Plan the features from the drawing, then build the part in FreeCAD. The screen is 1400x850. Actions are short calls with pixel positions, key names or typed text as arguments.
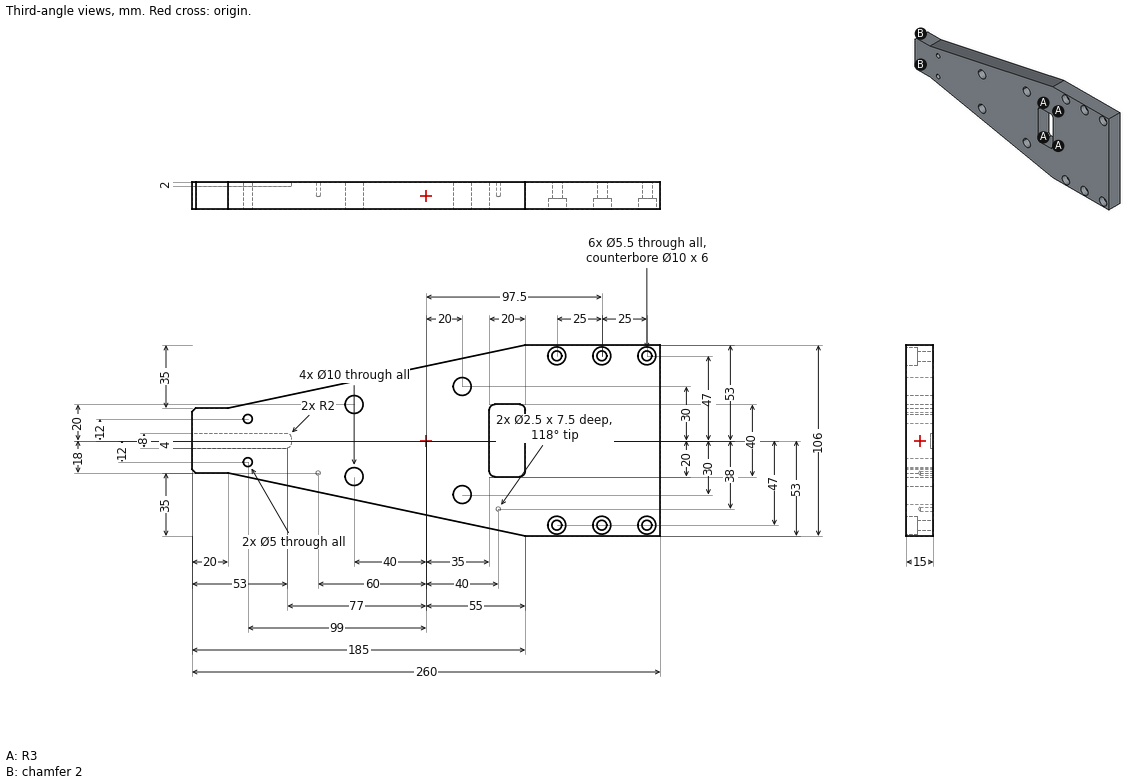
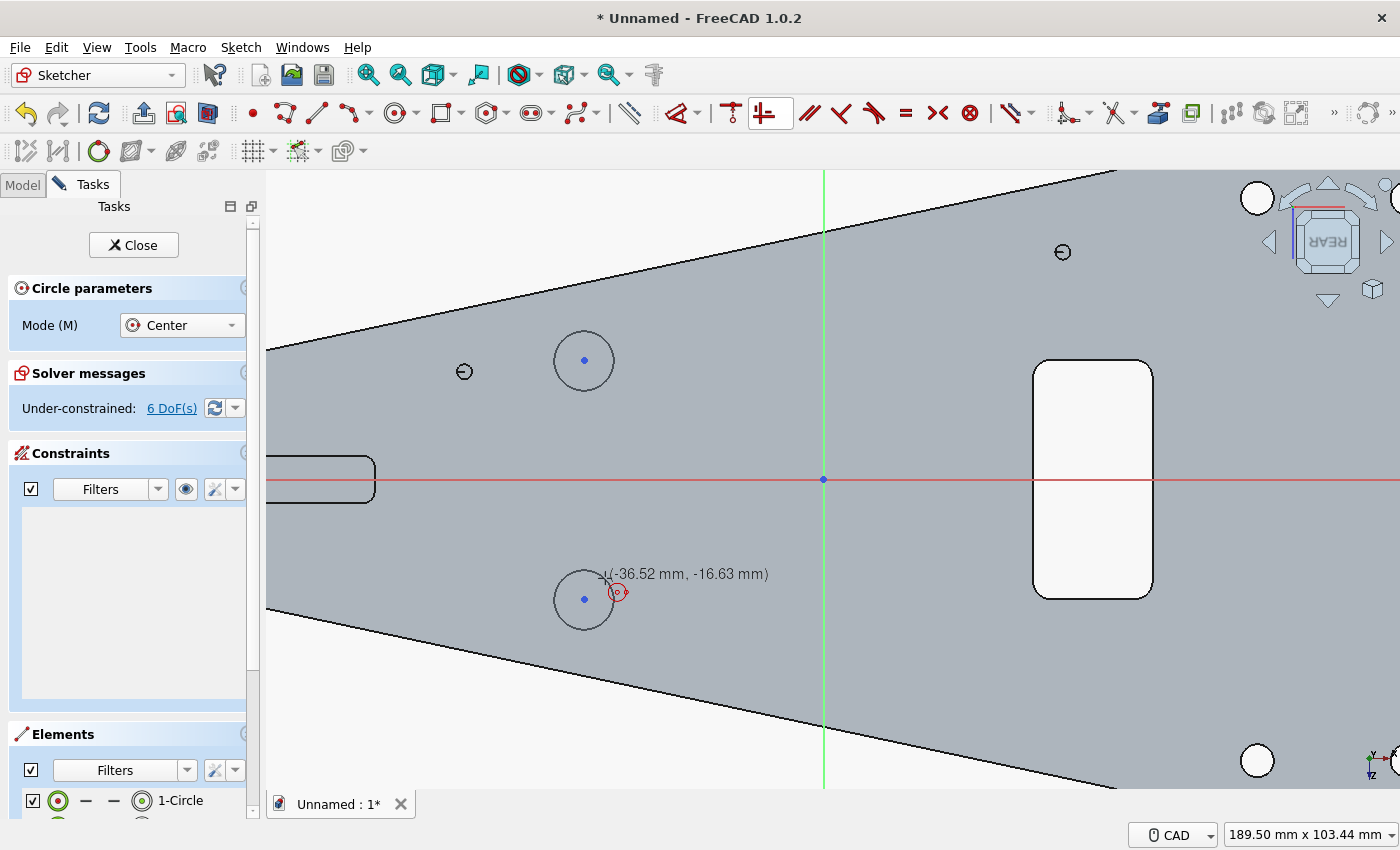
click(943, 659)
click(964, 638)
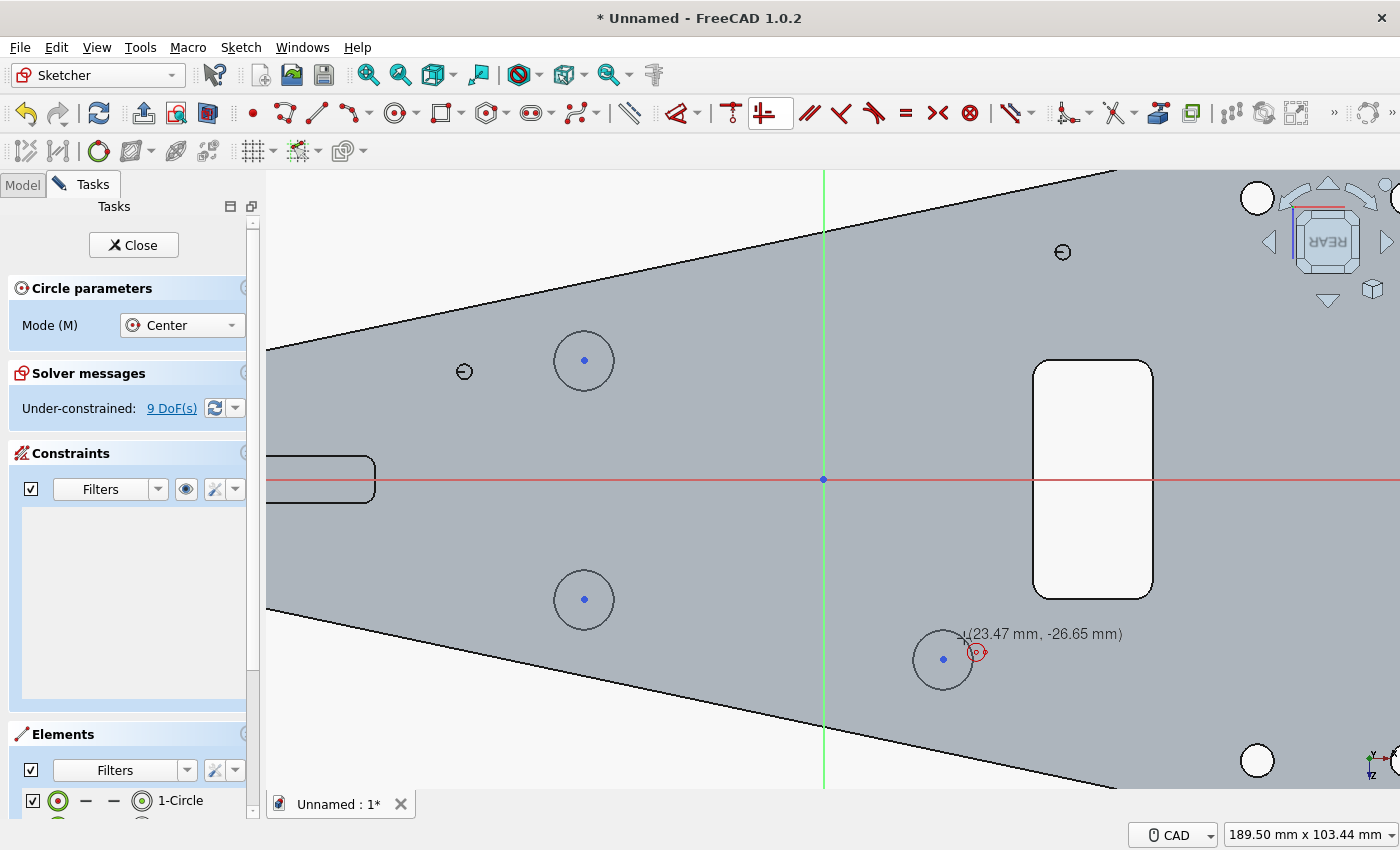
click(943, 300)
click(964, 279)
key(Escape)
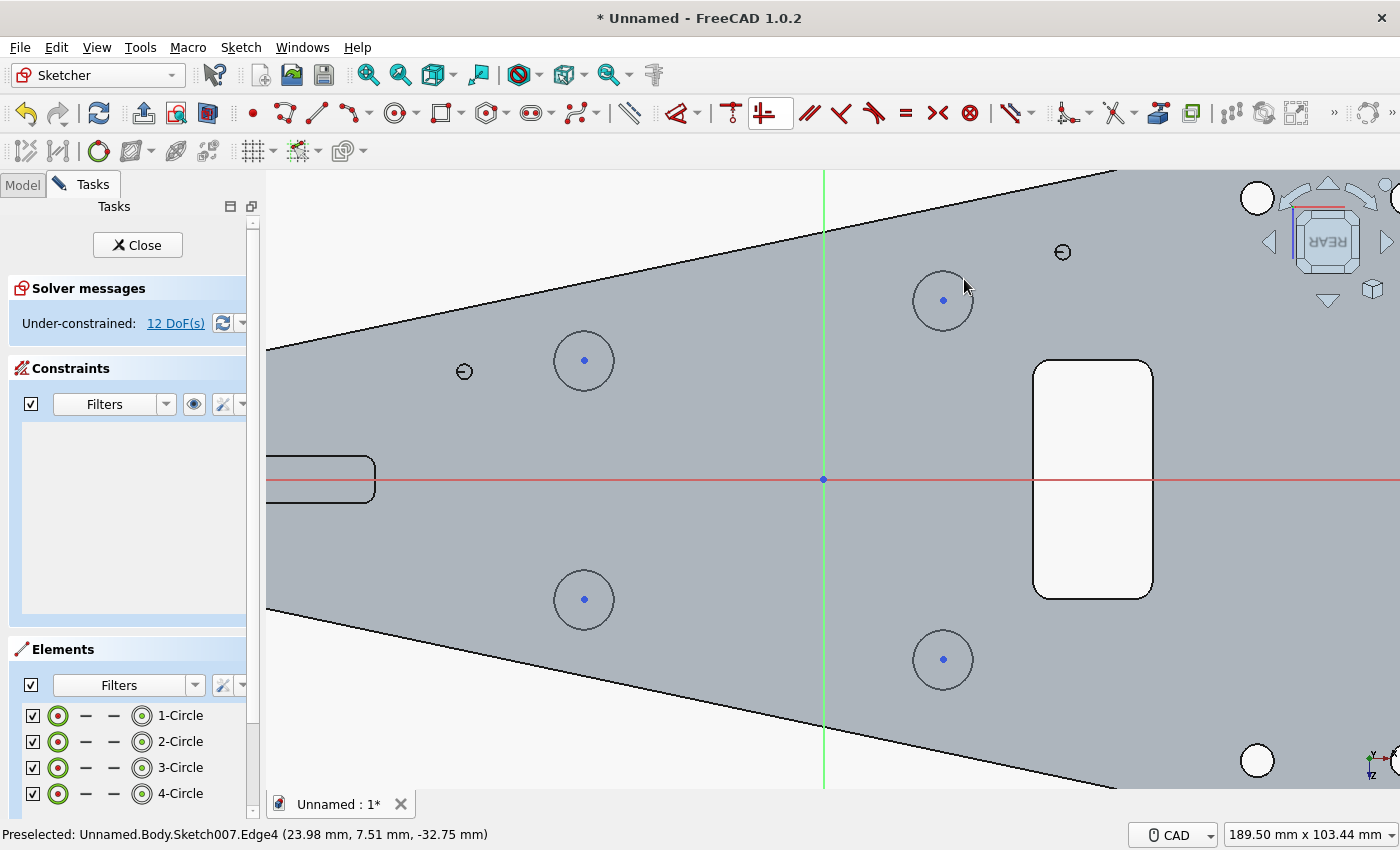
click(605, 340)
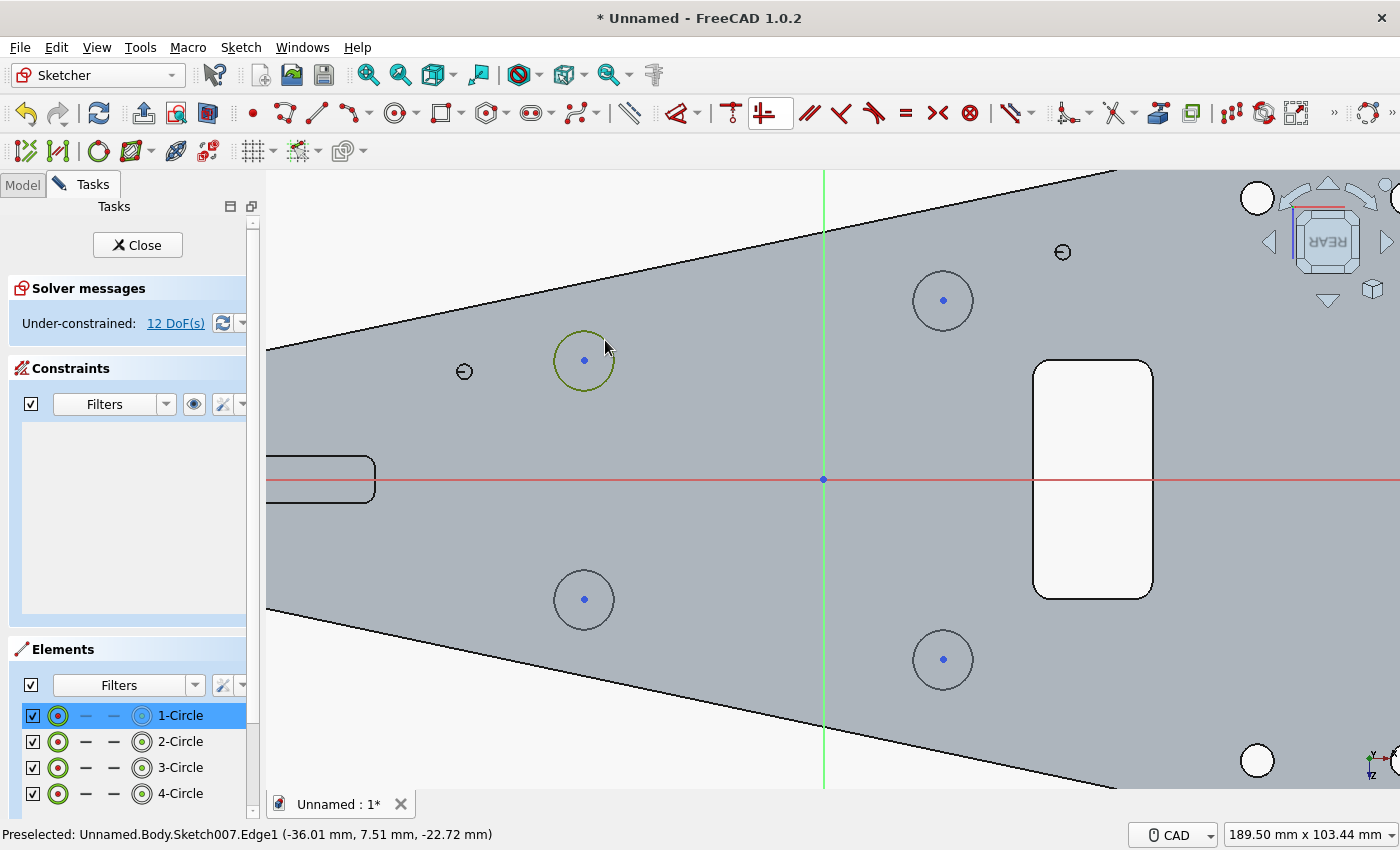
click(605, 579)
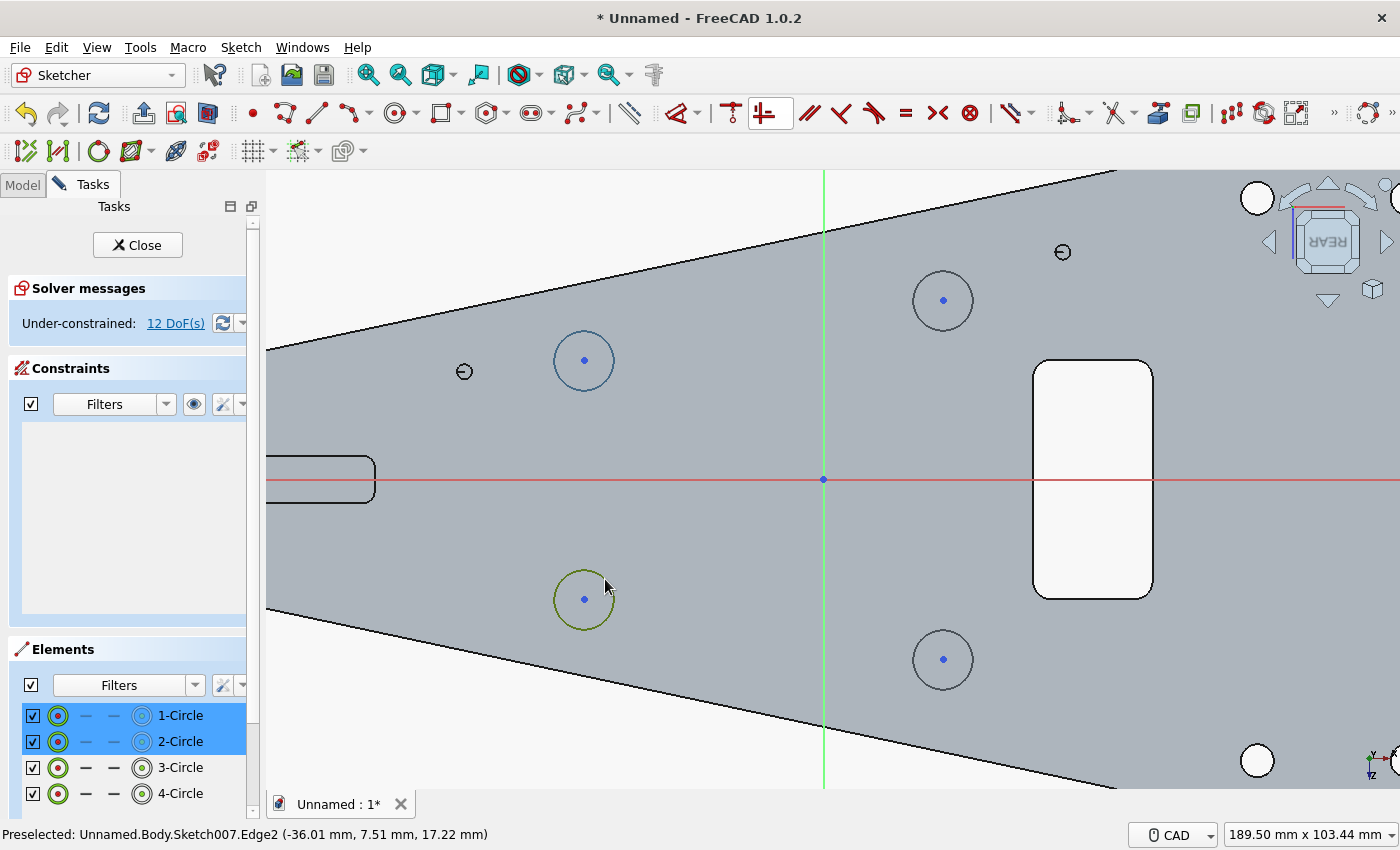
click(964, 639)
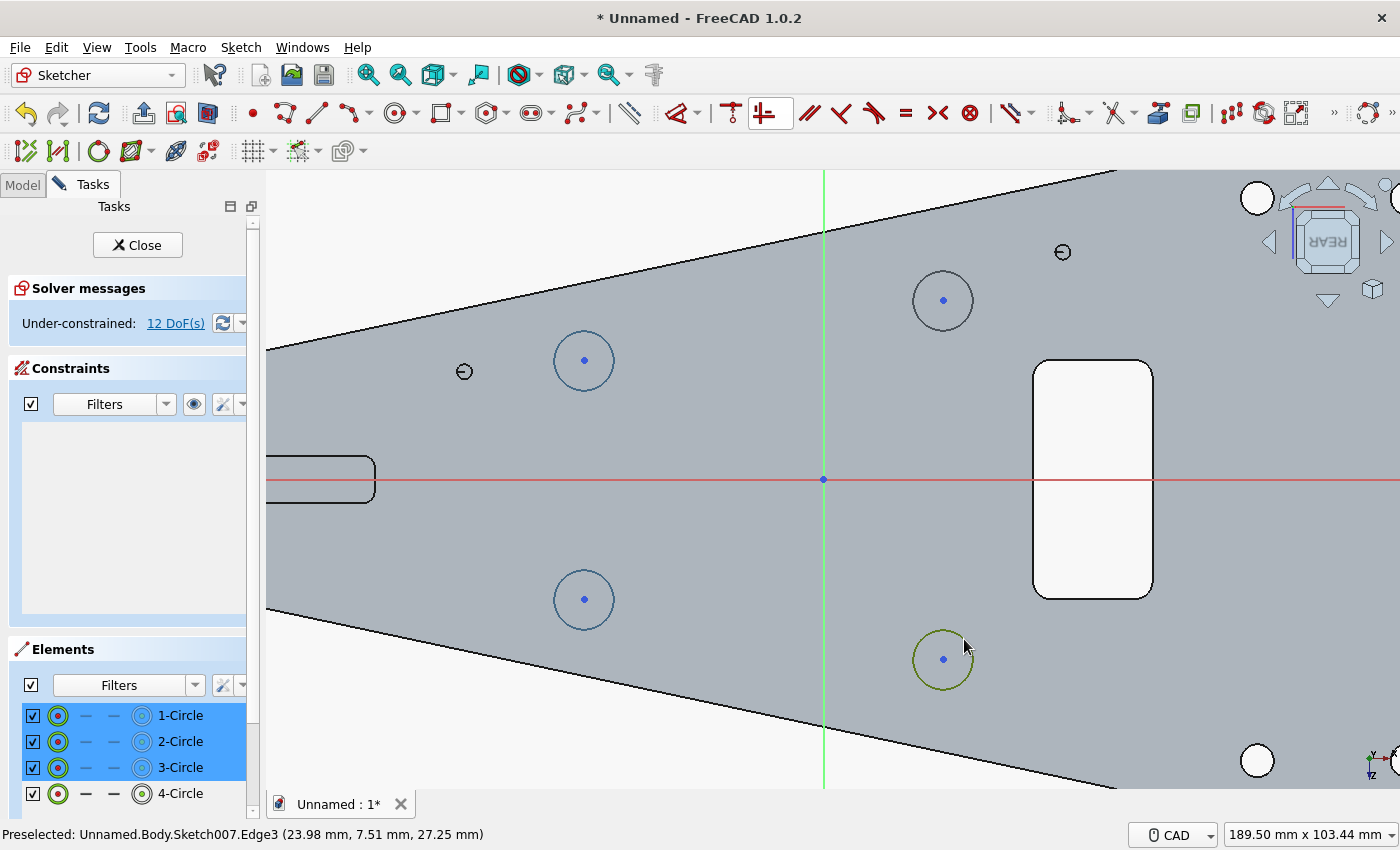
click(964, 280)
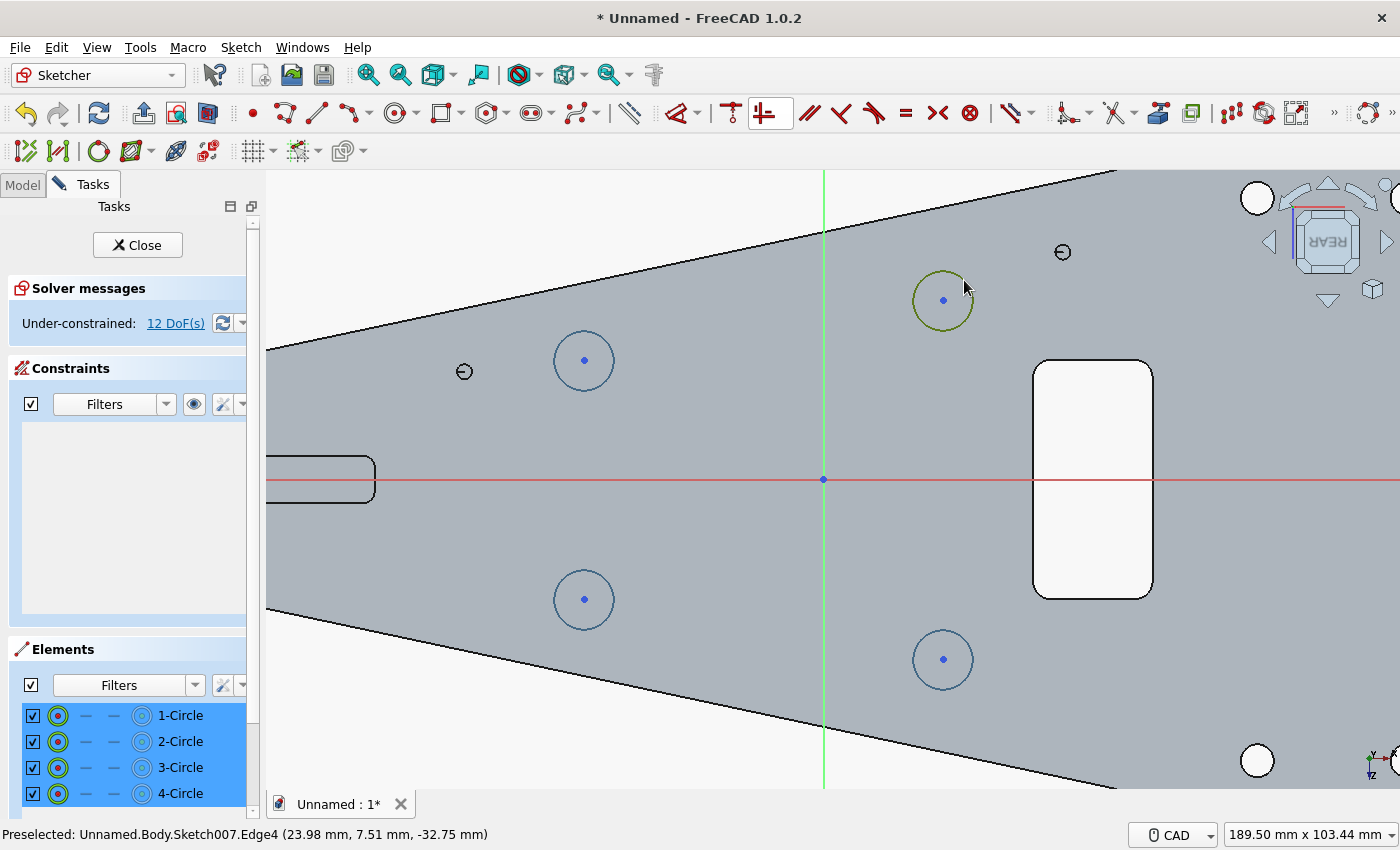
click(906, 114)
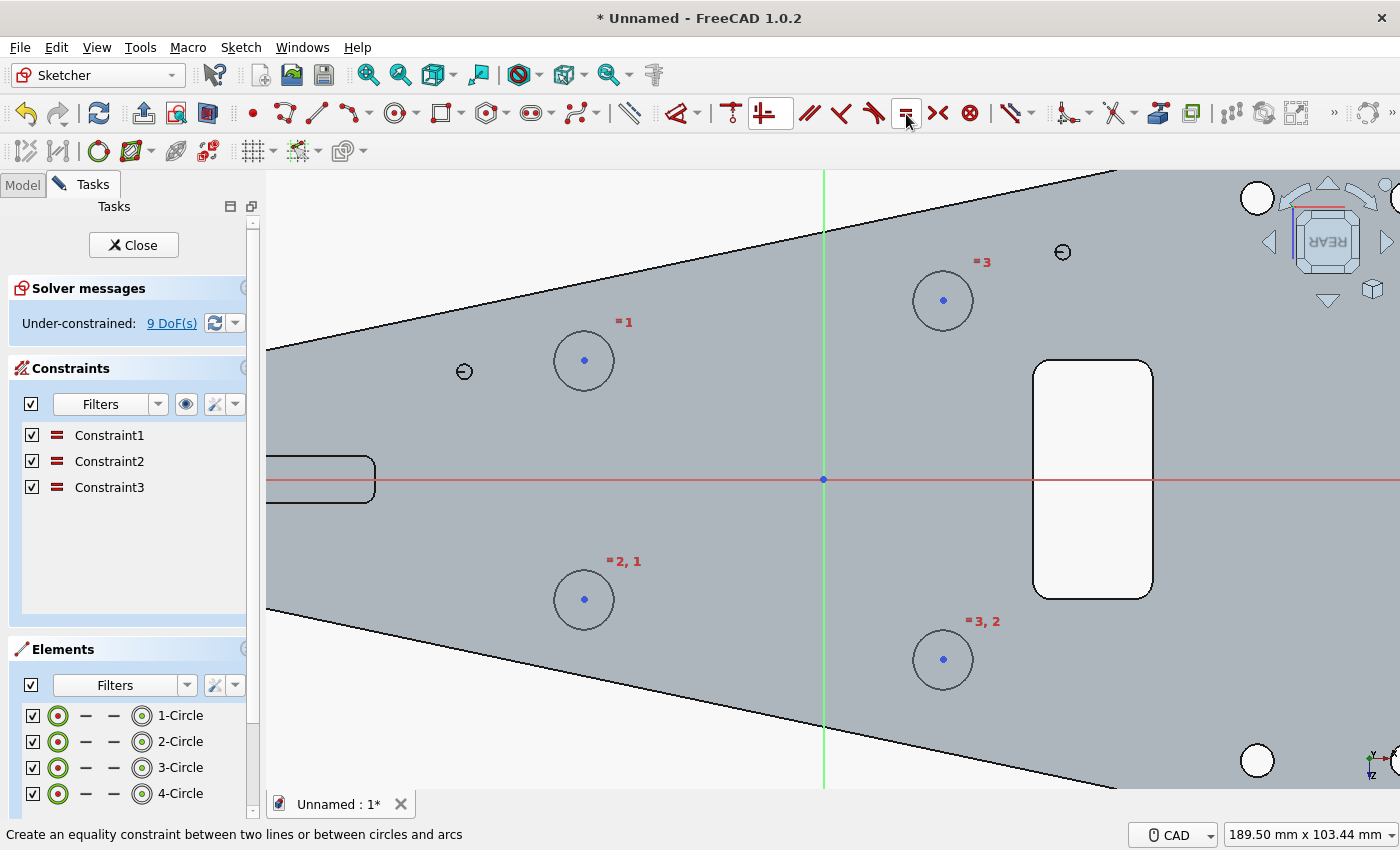
click(584, 361)